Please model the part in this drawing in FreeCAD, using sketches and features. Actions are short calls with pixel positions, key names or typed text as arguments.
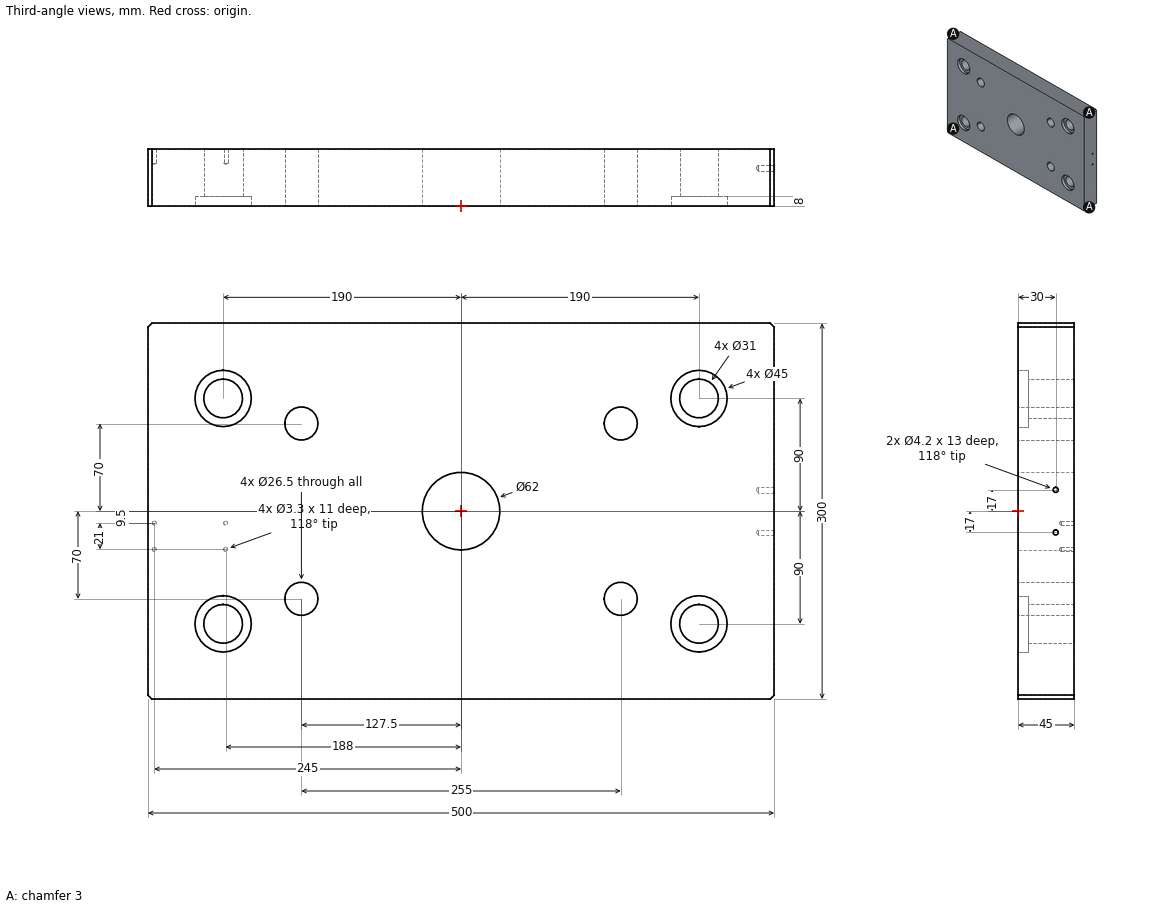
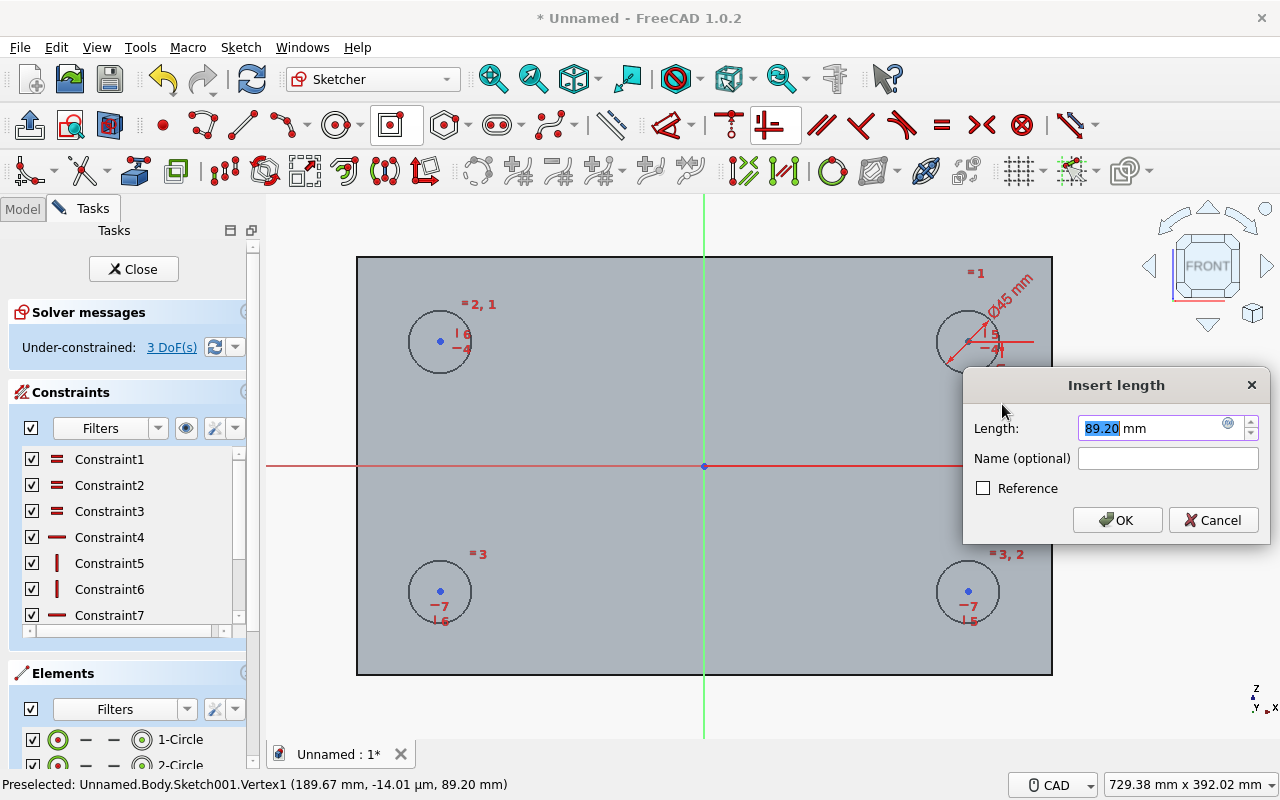
text(90)
key(Return)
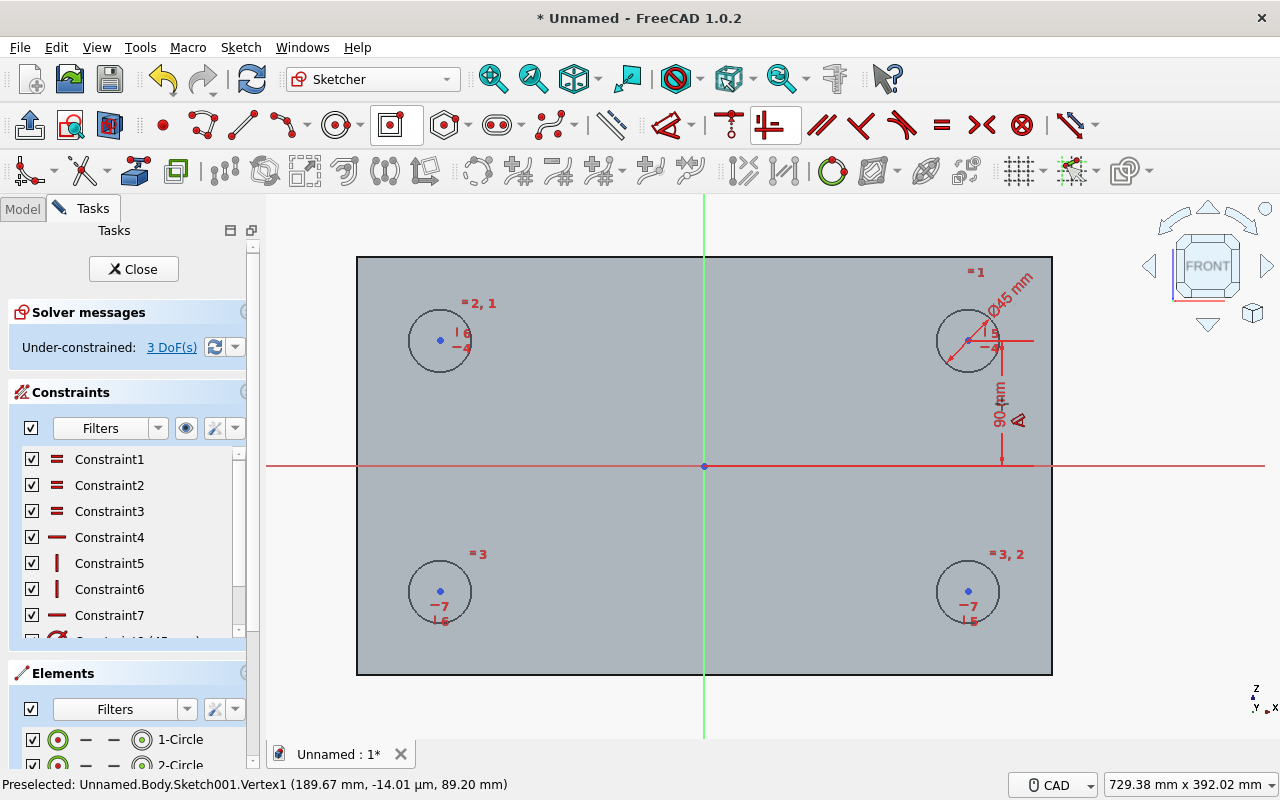
click(968, 592)
click(1002, 529)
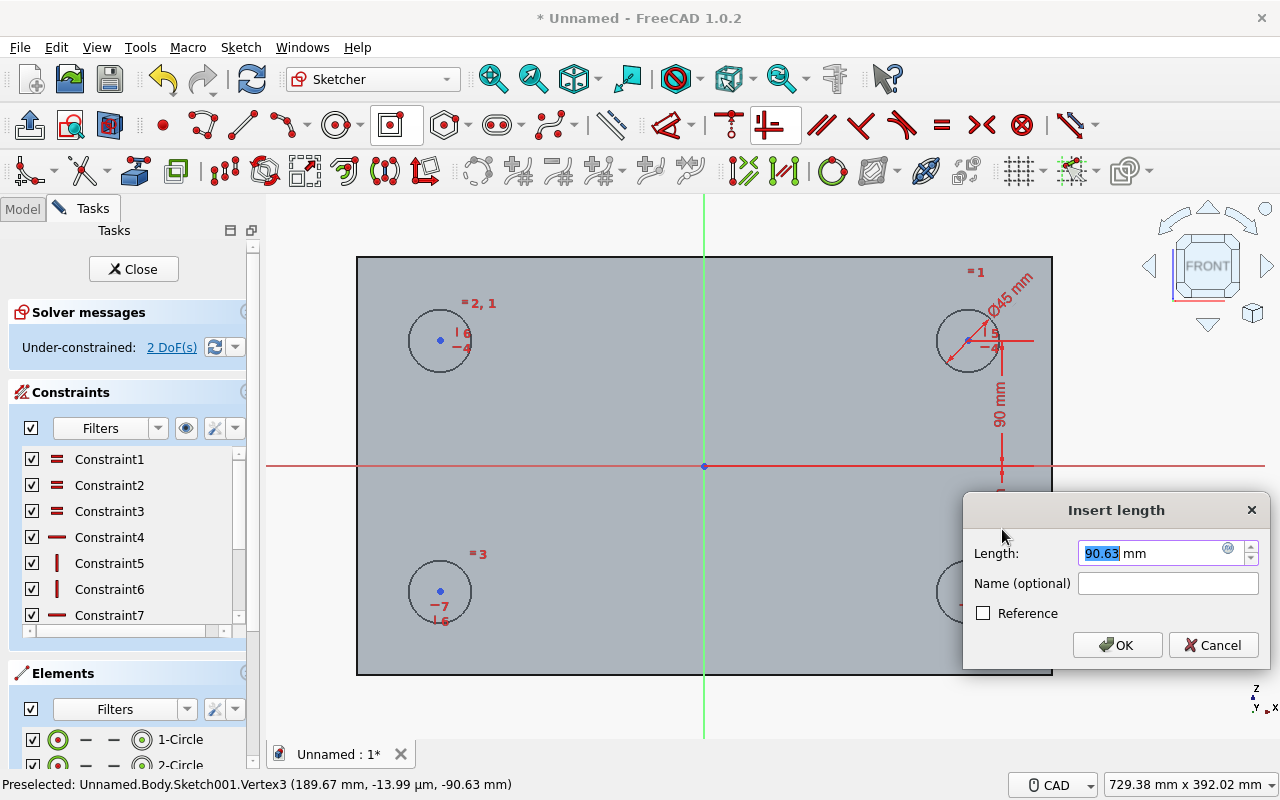
text(90)
key(Return)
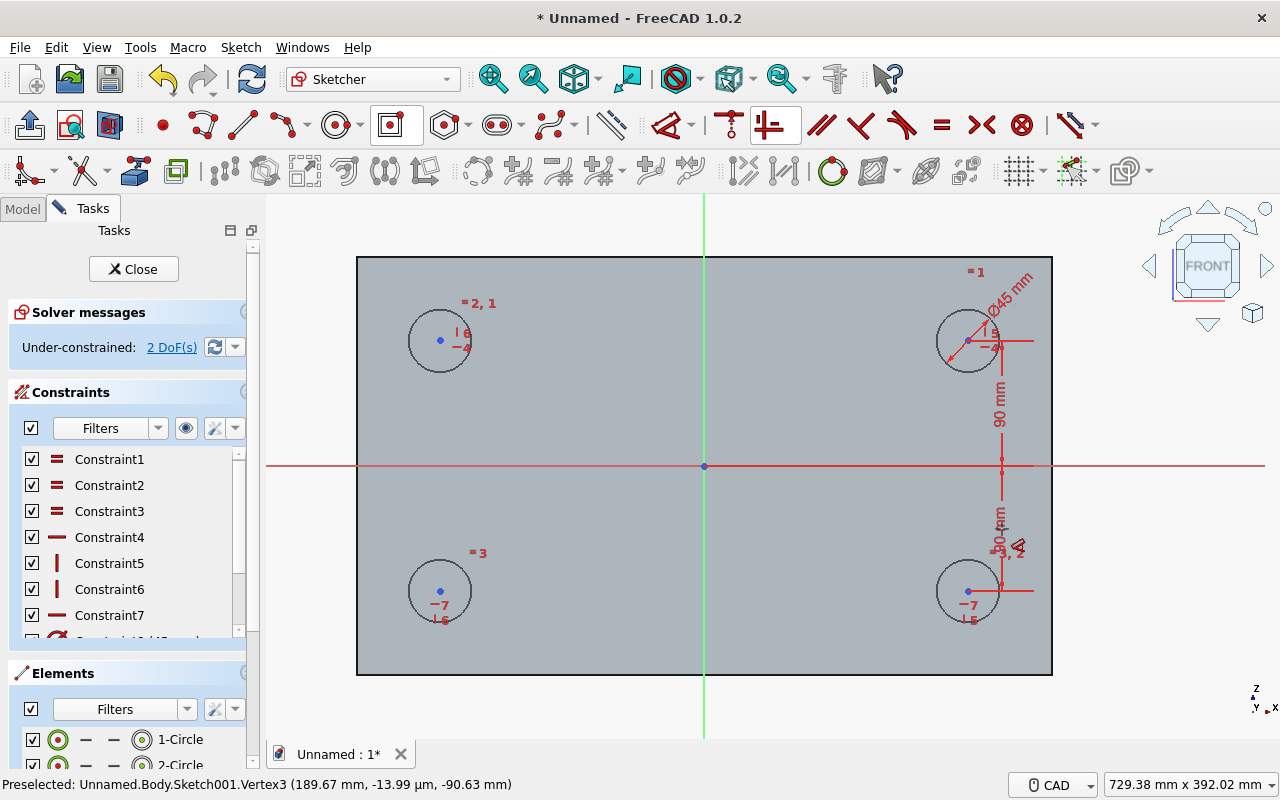
click(968, 341)
click(836, 307)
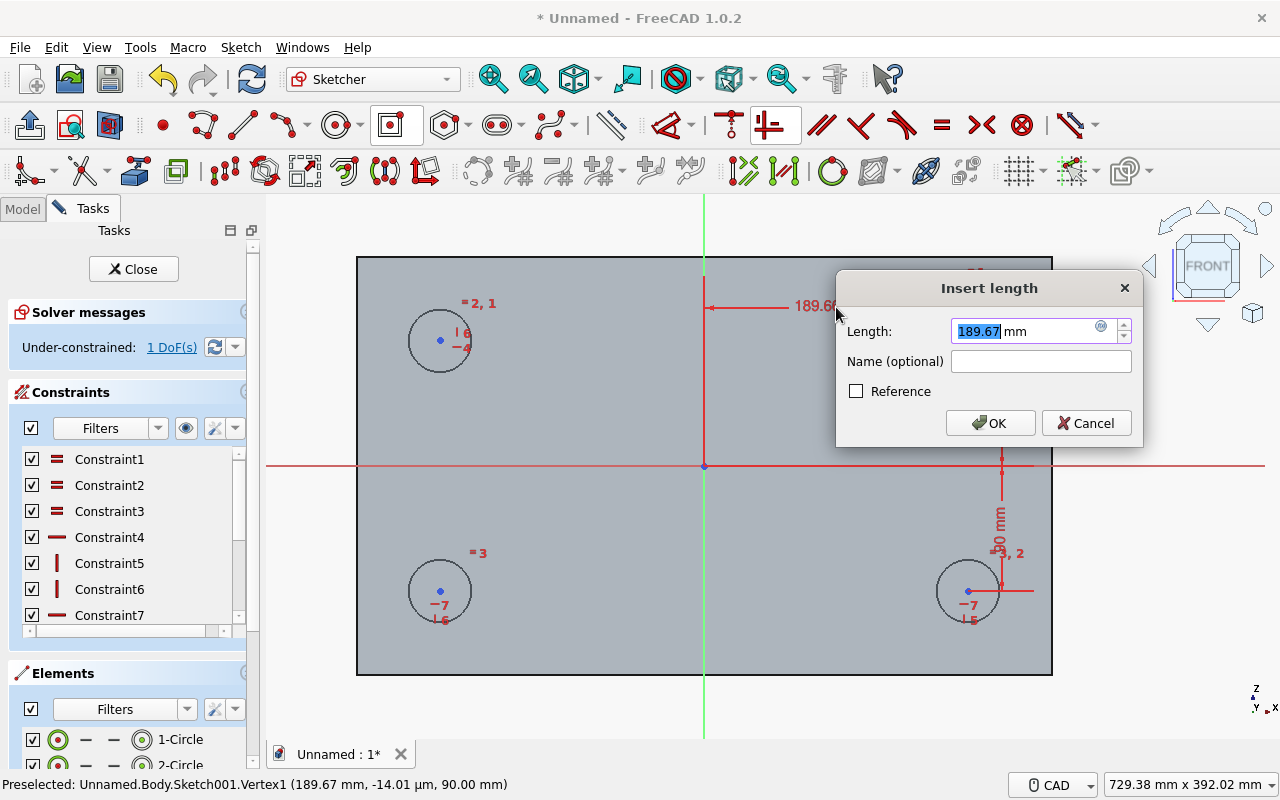
text(190)
key(Return)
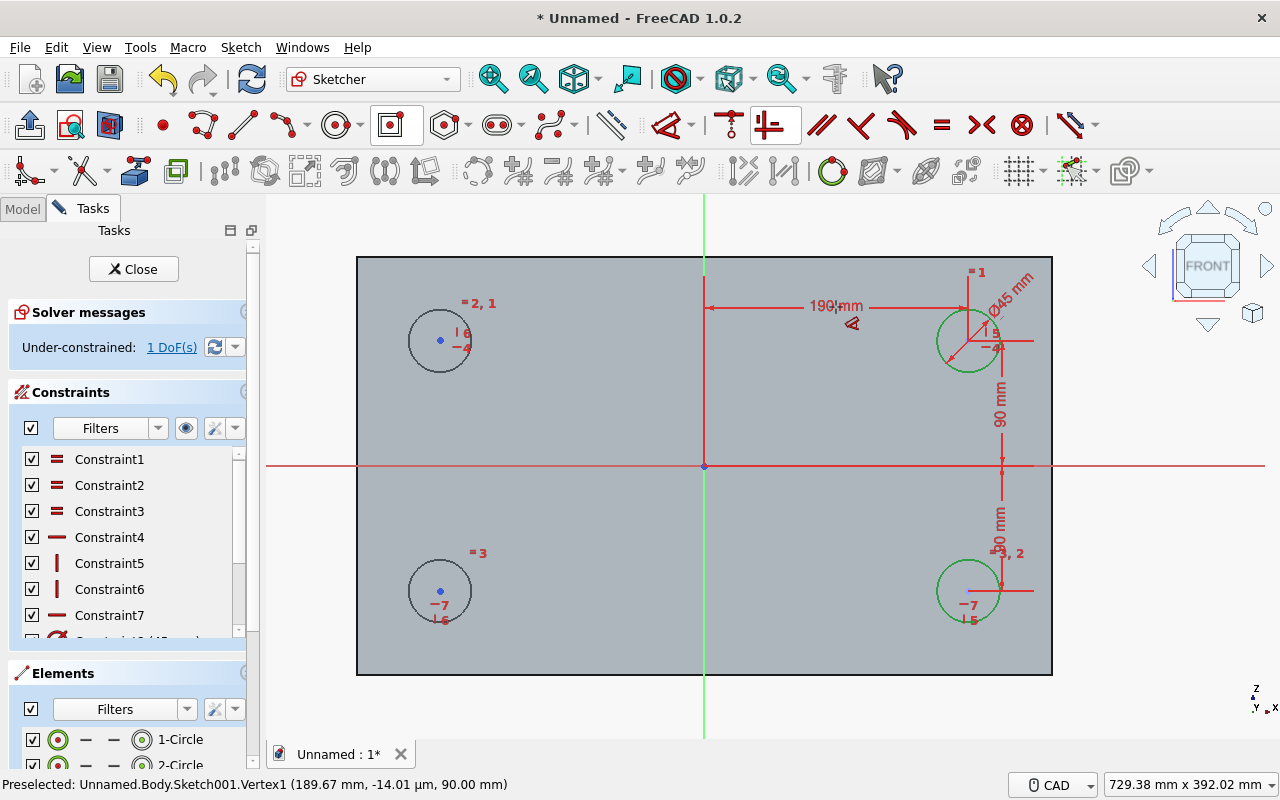
click(440, 341)
click(572, 307)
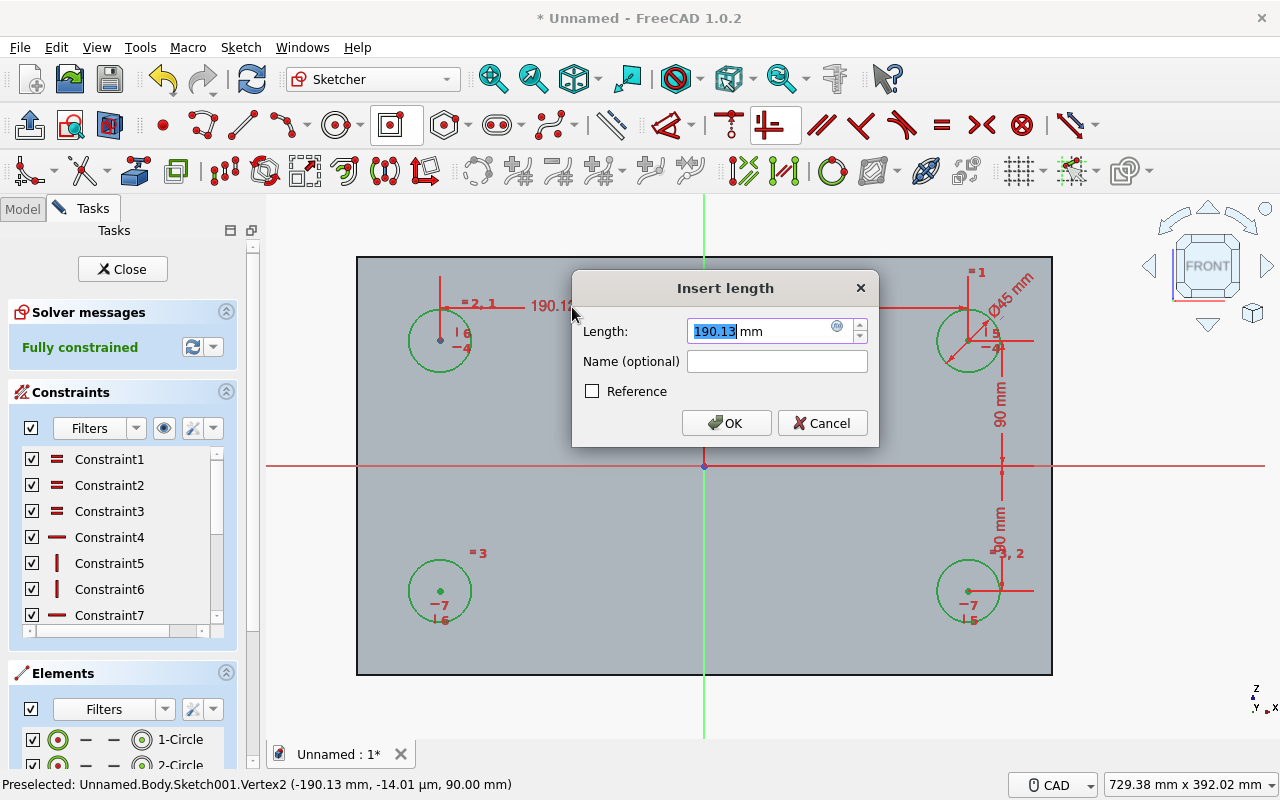
text(190)
key(Return)
key(Escape)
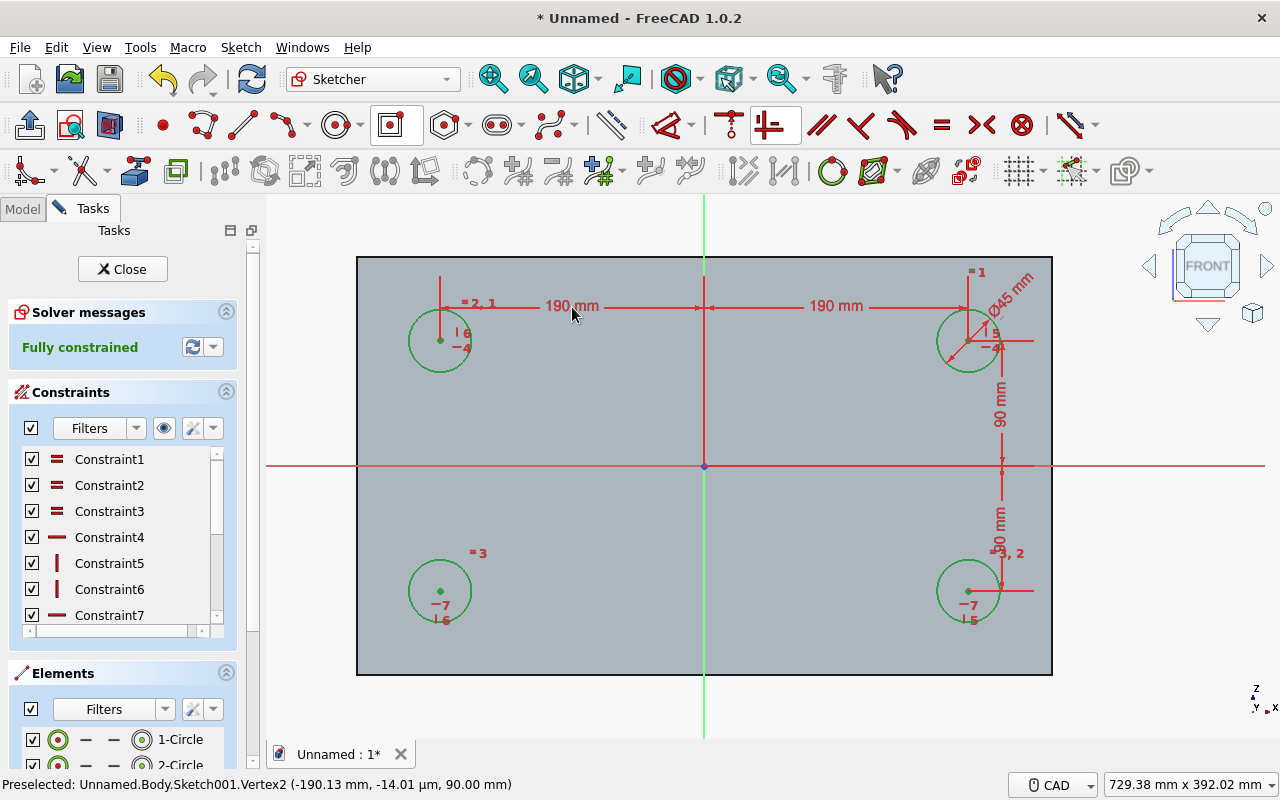
click(123, 269)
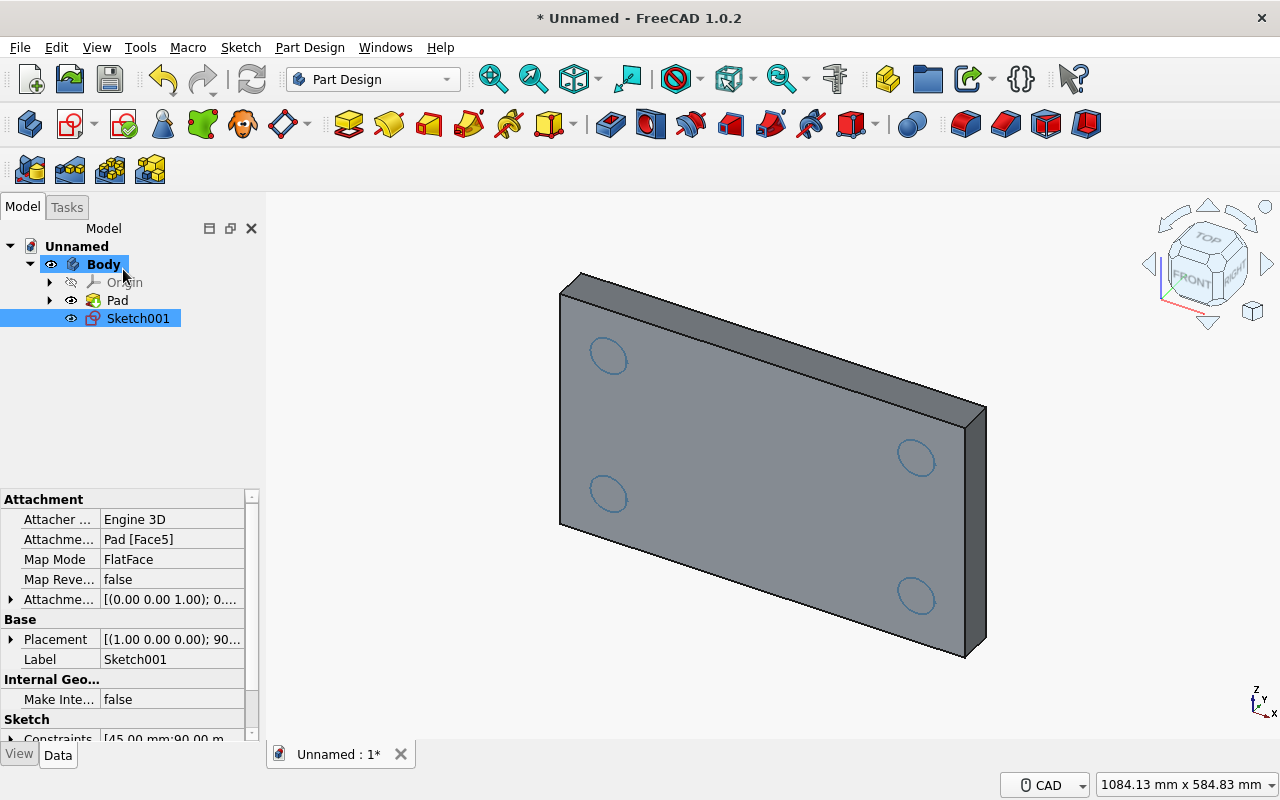
click(612, 124)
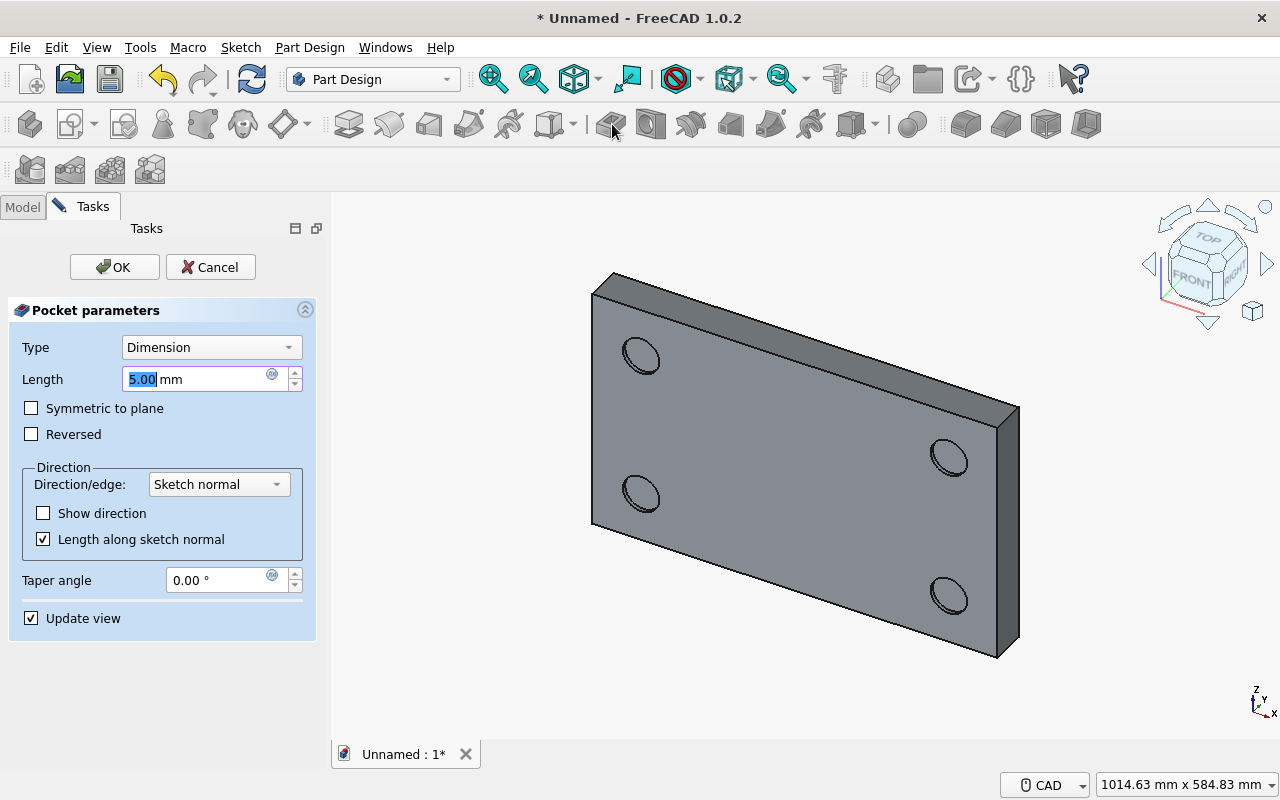
text(8)
key(Tab)